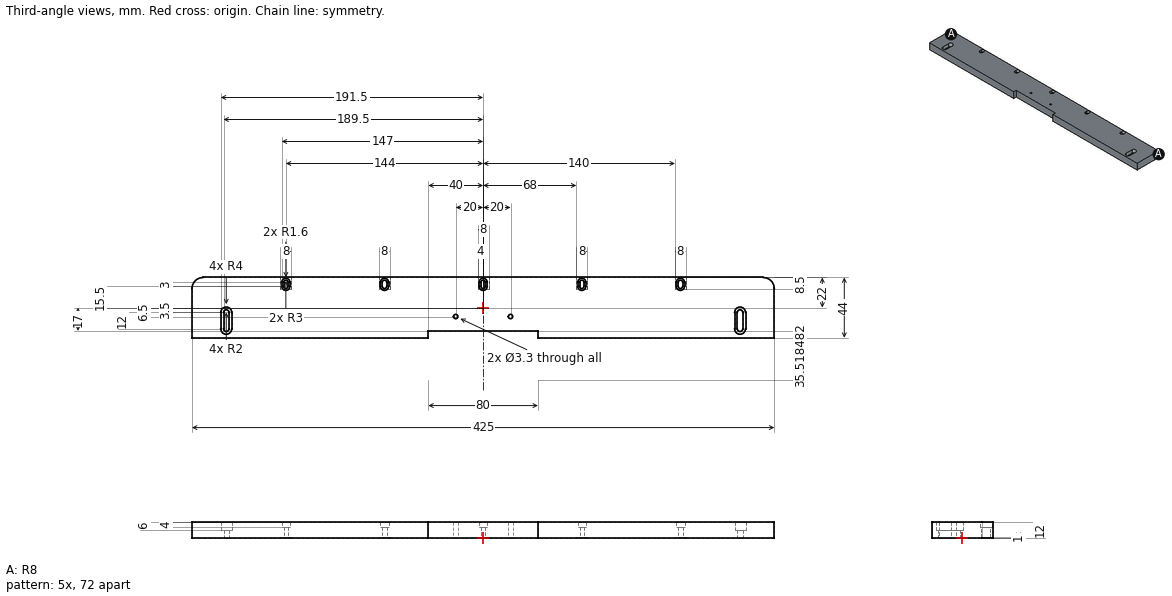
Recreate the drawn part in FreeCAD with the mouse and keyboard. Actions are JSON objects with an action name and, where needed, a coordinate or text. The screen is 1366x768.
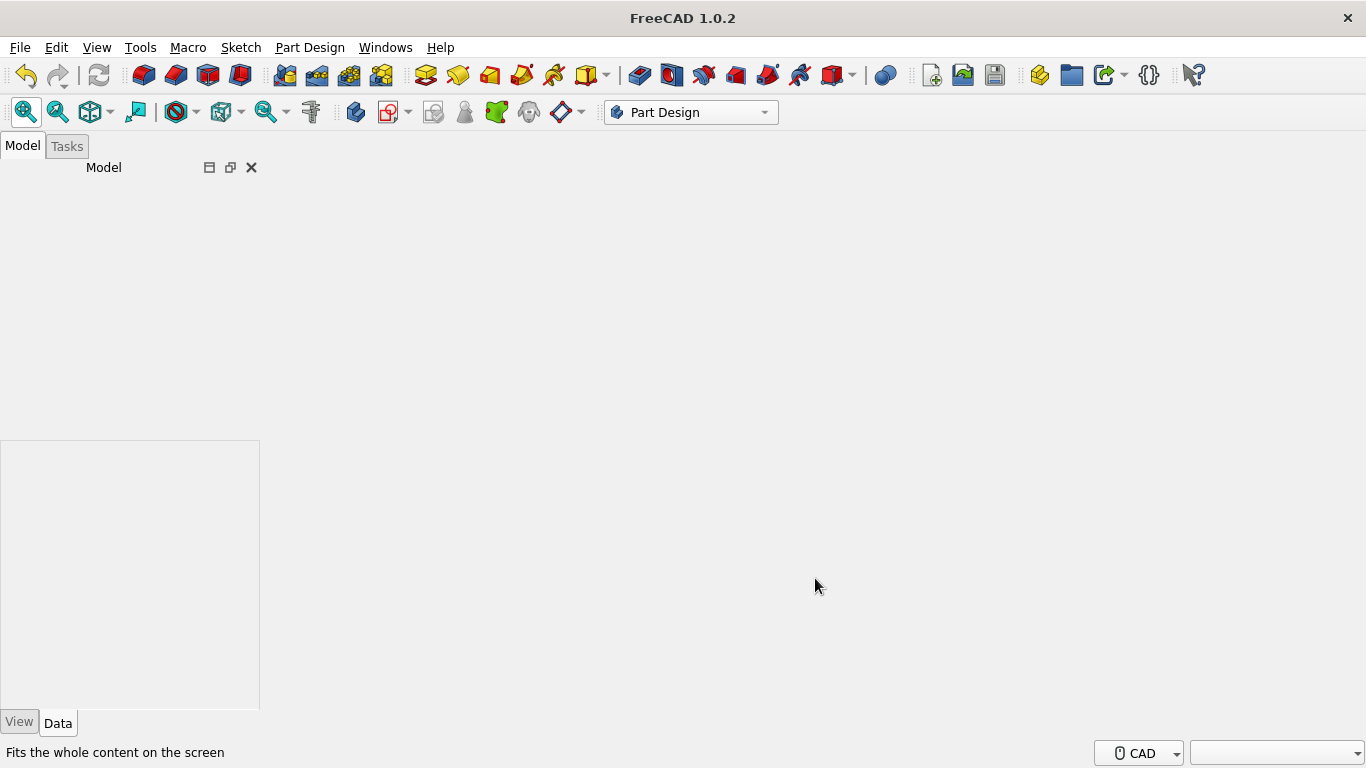
{"action": "left_click", "coordinate": [932, 76]}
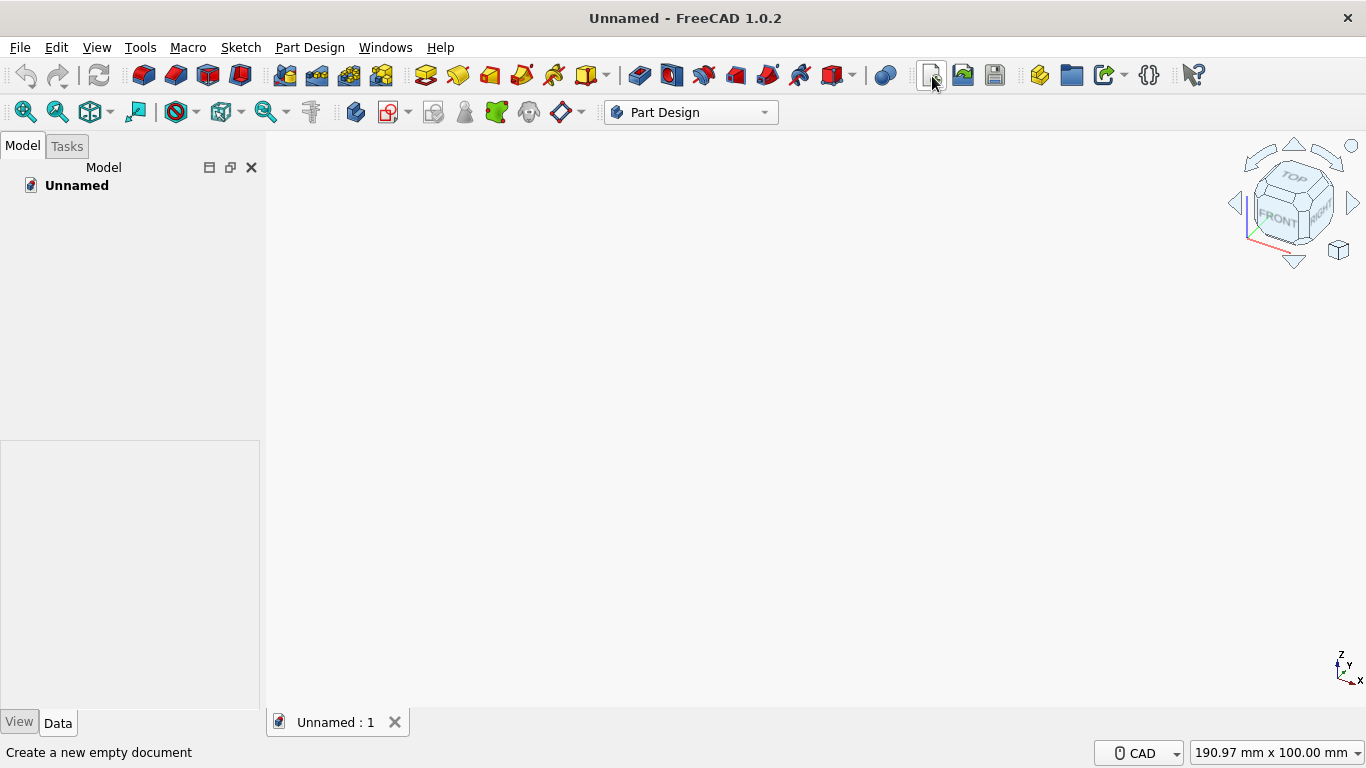
{"action": "left_click", "coordinate": [388, 112]}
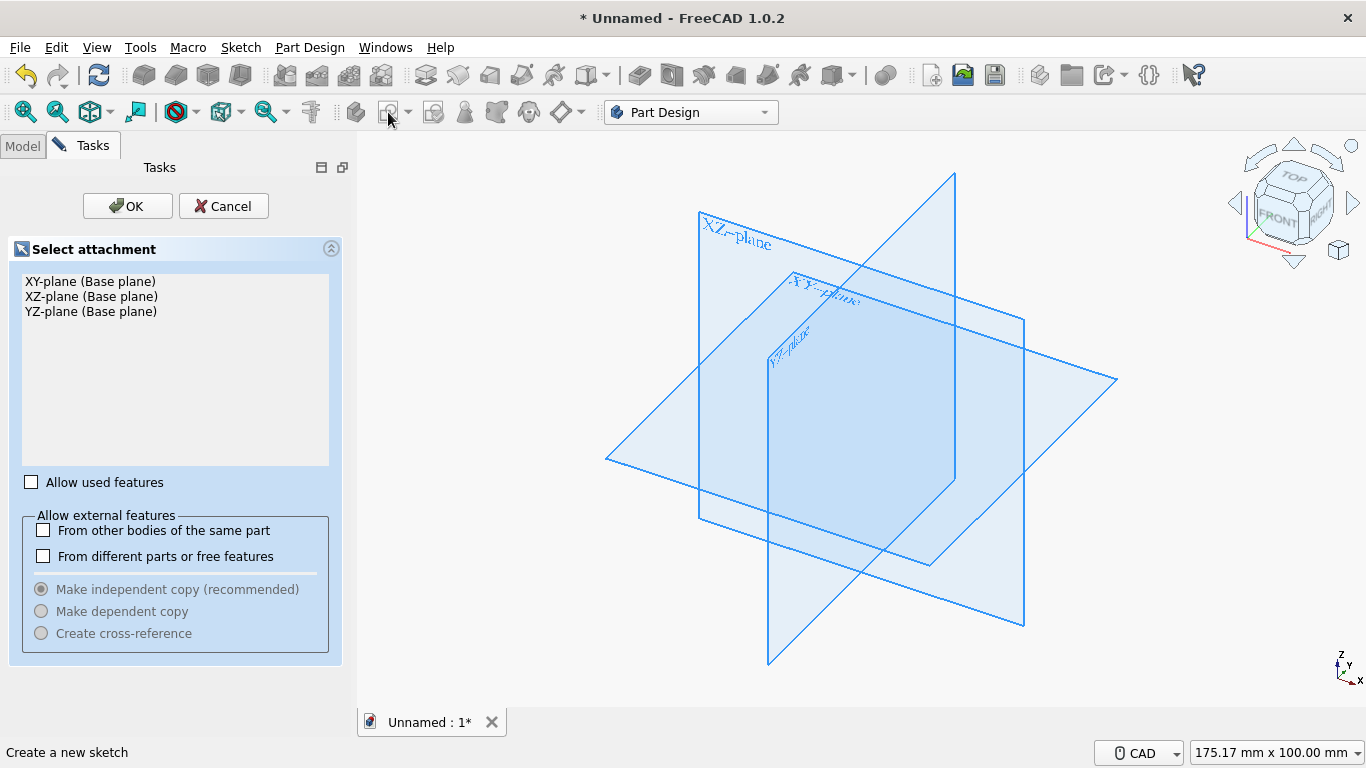
{"action": "left_click", "coordinate": [82, 282]}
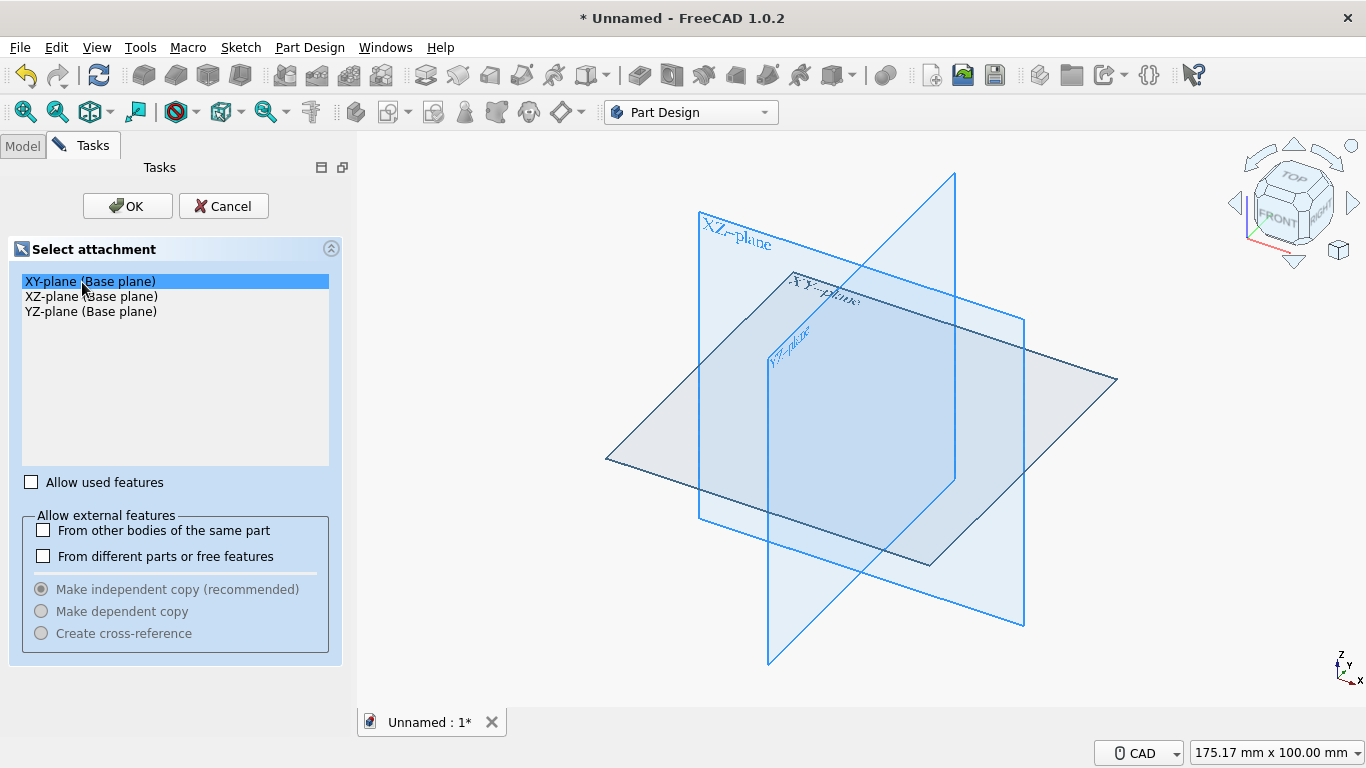
{"action": "left_click", "coordinate": [128, 206]}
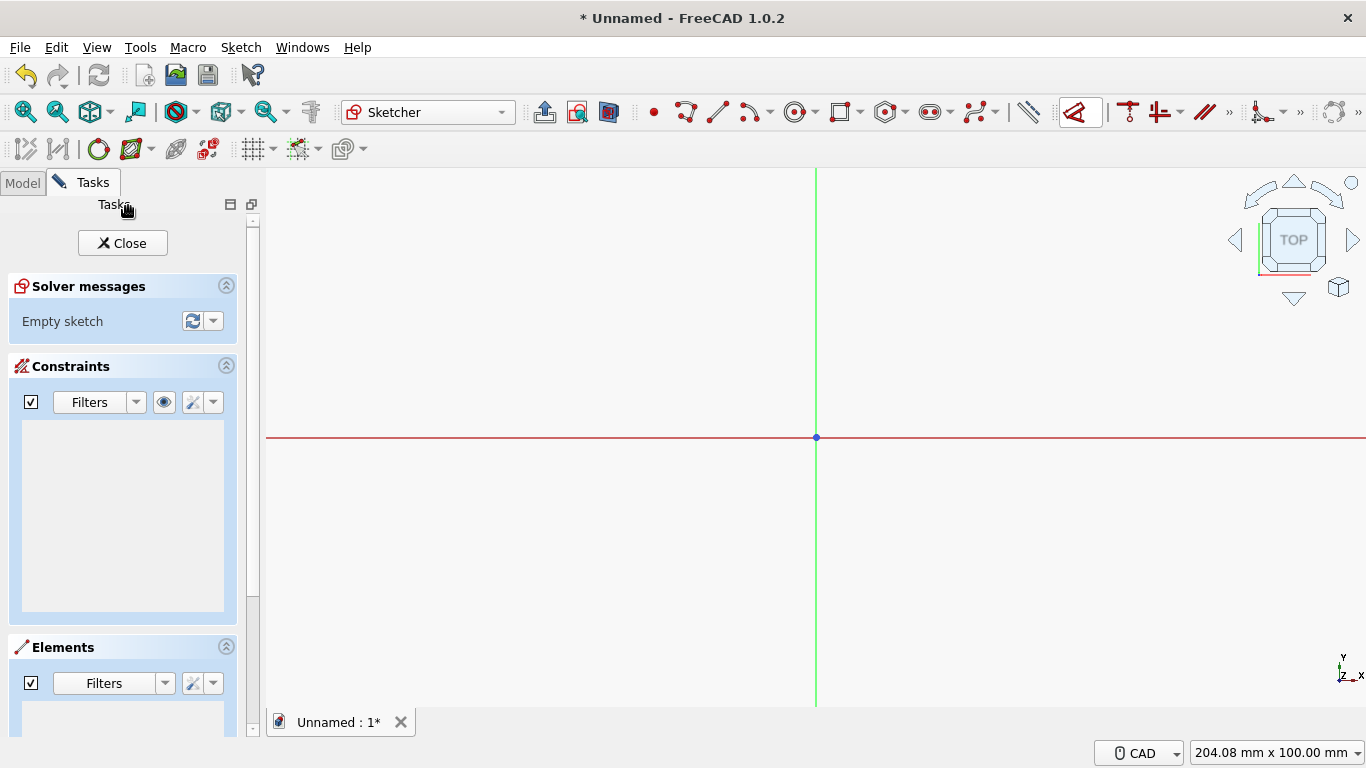
{"action": "scroll", "coordinate": [718, 438], "scroll_direction": "down", "scroll_amount": 6}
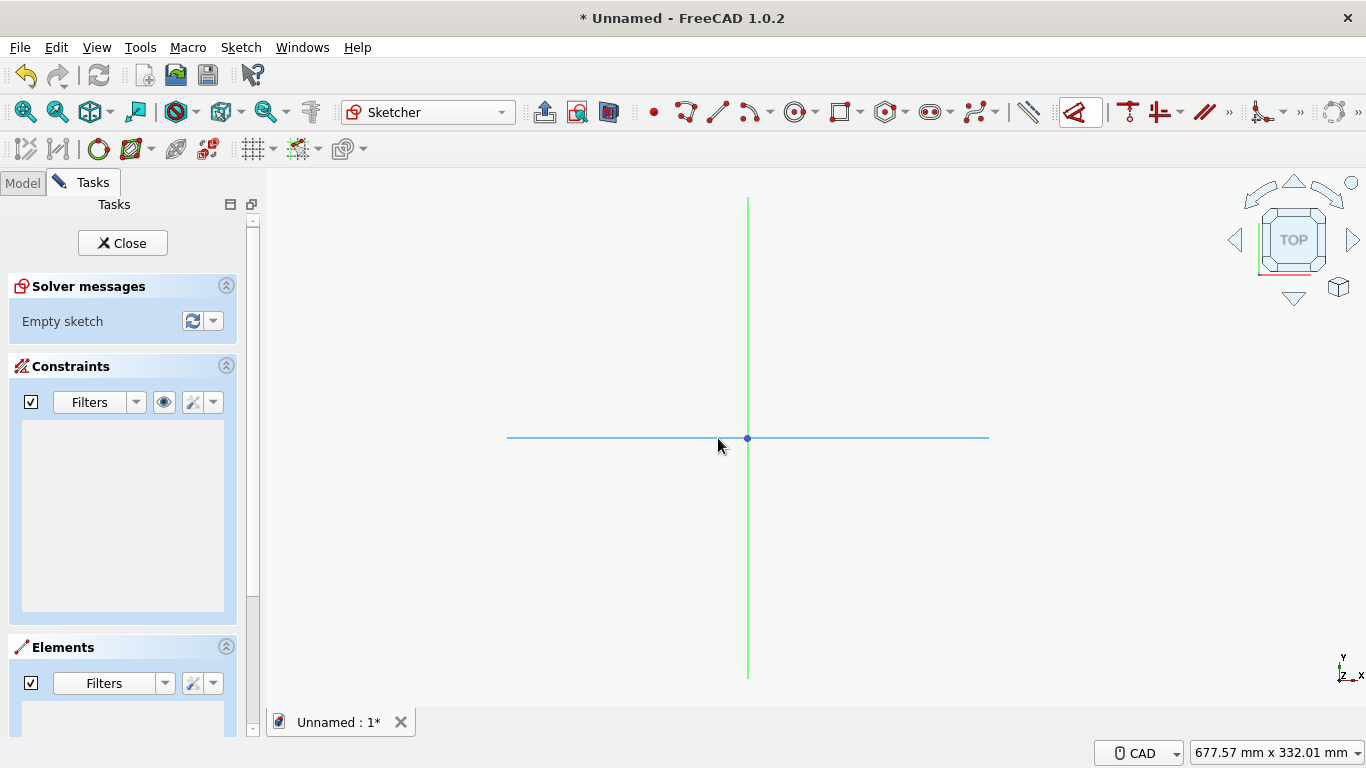
{"action": "key", "text": "g v"}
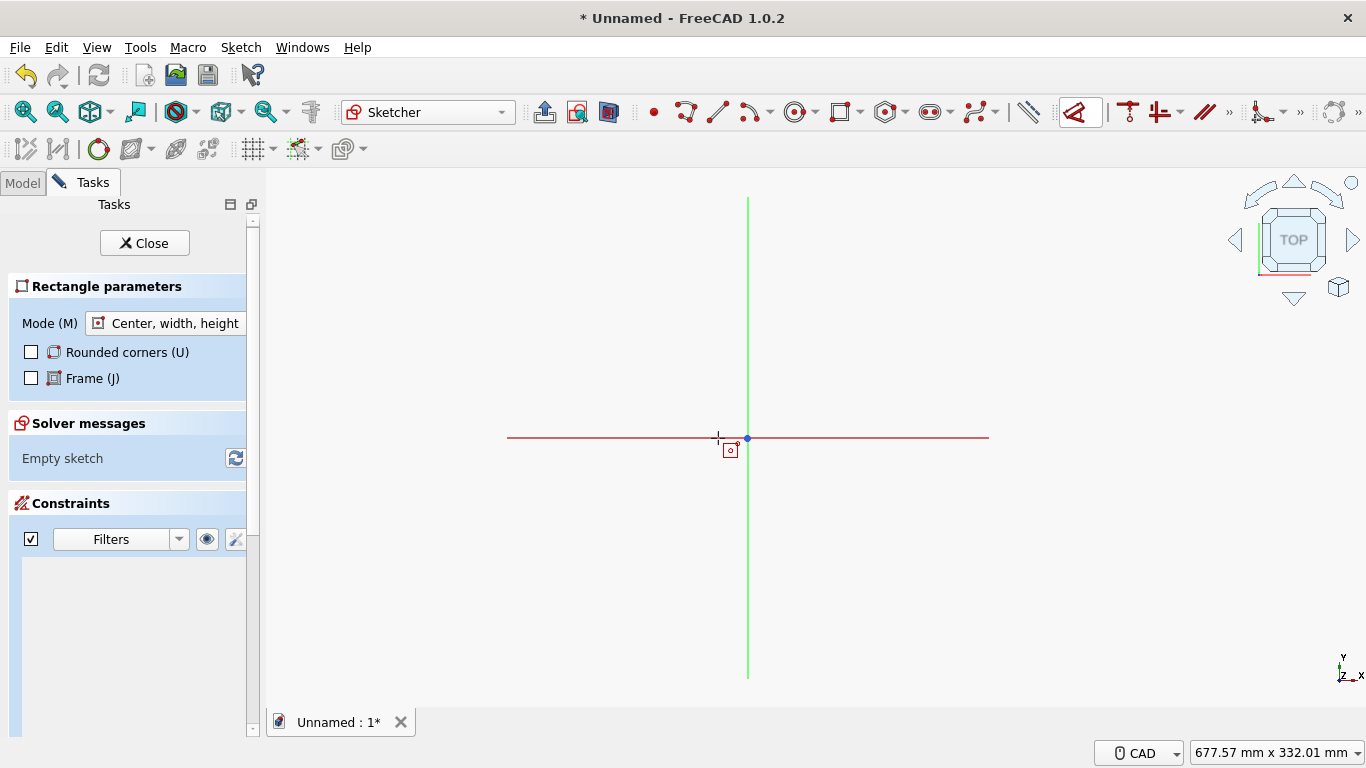
{"action": "left_click", "coordinate": [748, 438]}
{"action": "mouse_move", "coordinate": [1093, 402]}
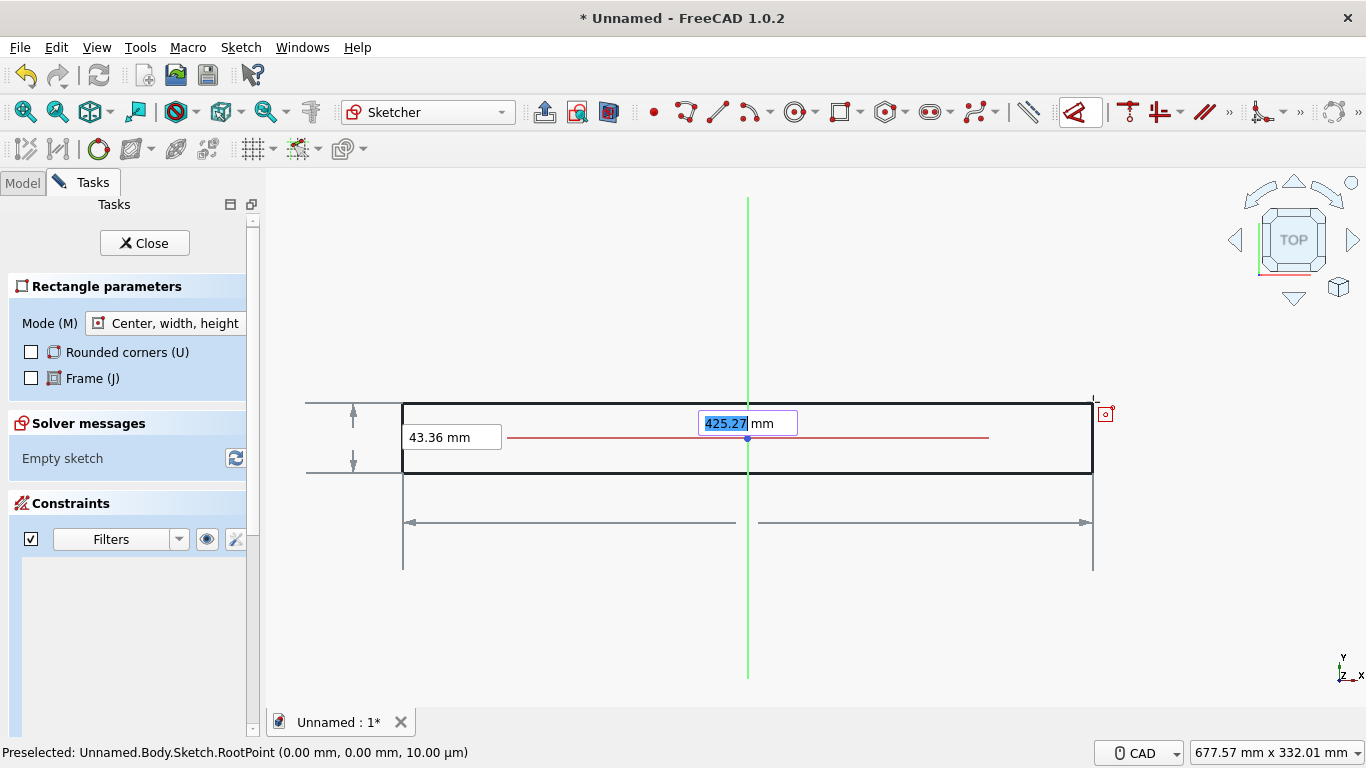
{"action": "type", "text": "425"}
{"action": "key", "text": "Tab"}
{"action": "type", "text": "44"}
{"action": "key", "text": "Return"}
{"action": "key", "text": "Escape"}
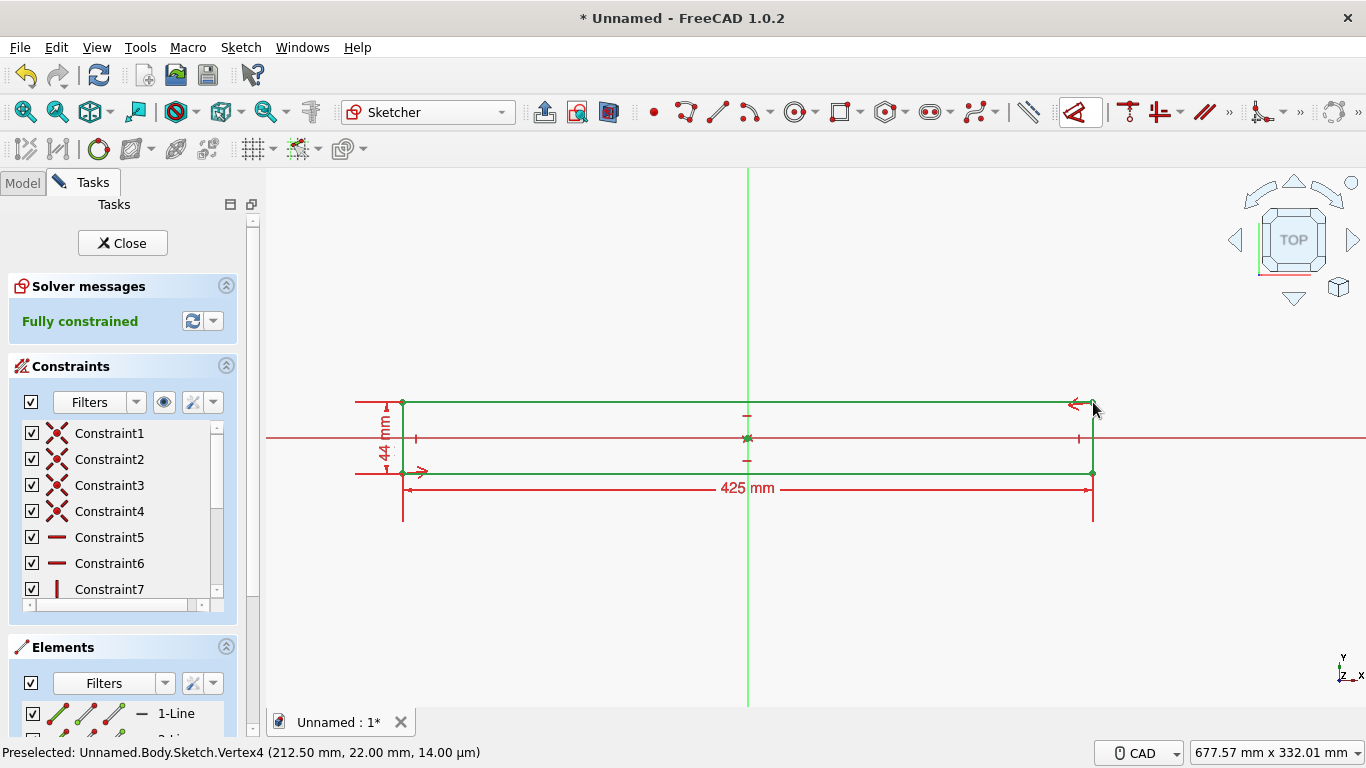
{"action": "left_click", "coordinate": [123, 243]}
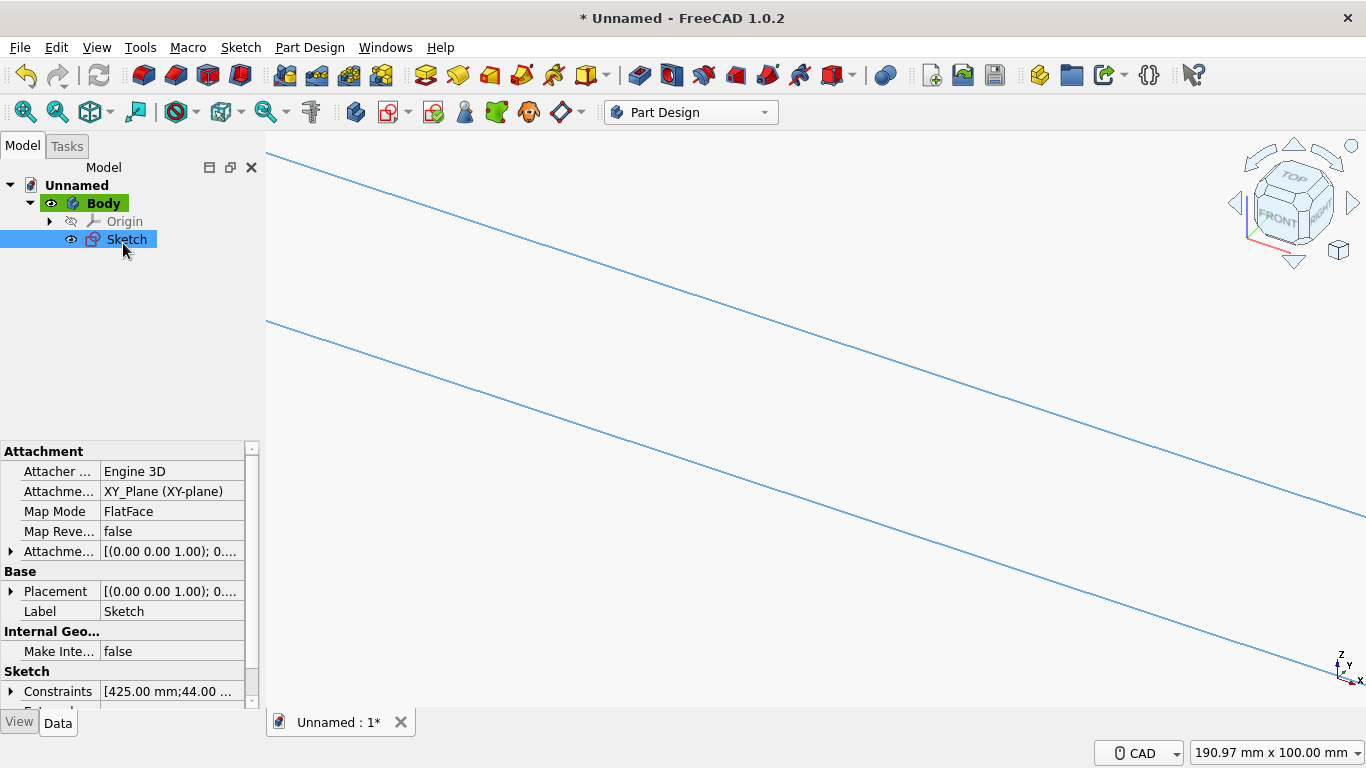
{"action": "left_click", "coordinate": [426, 76]}